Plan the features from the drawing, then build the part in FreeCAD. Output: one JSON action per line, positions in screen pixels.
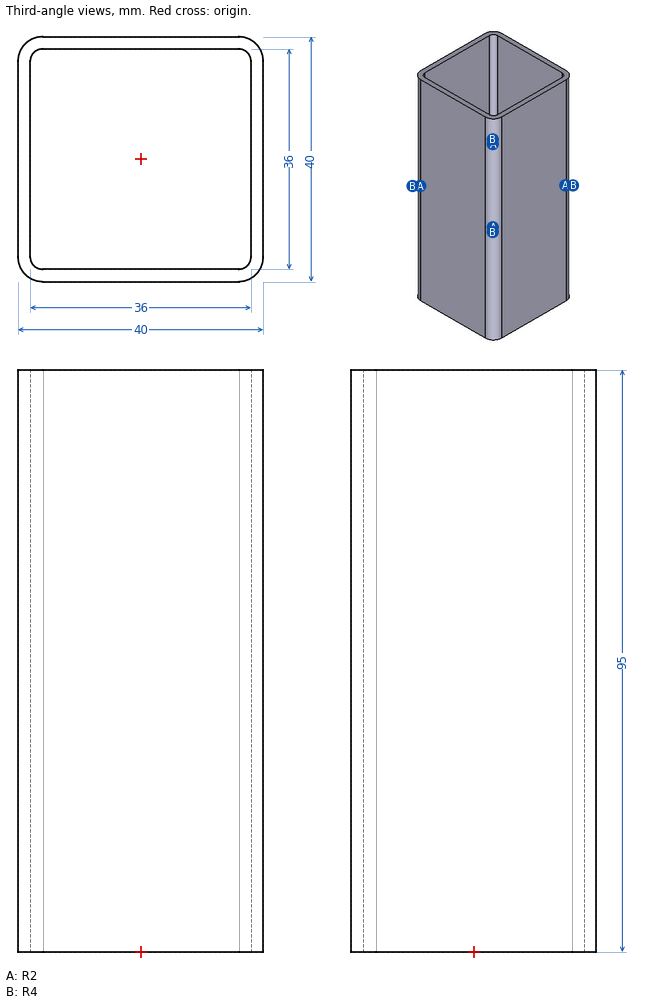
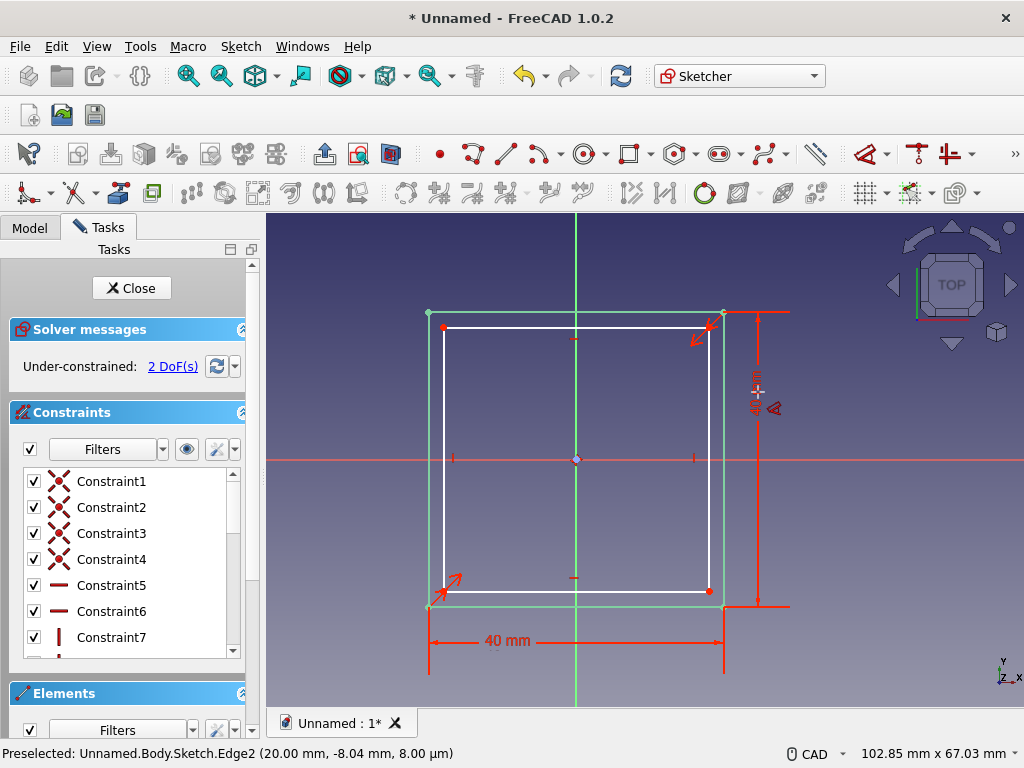
{"action": "left_click", "coordinate": [523, 592]}
{"action": "left_click", "coordinate": [637, 626]}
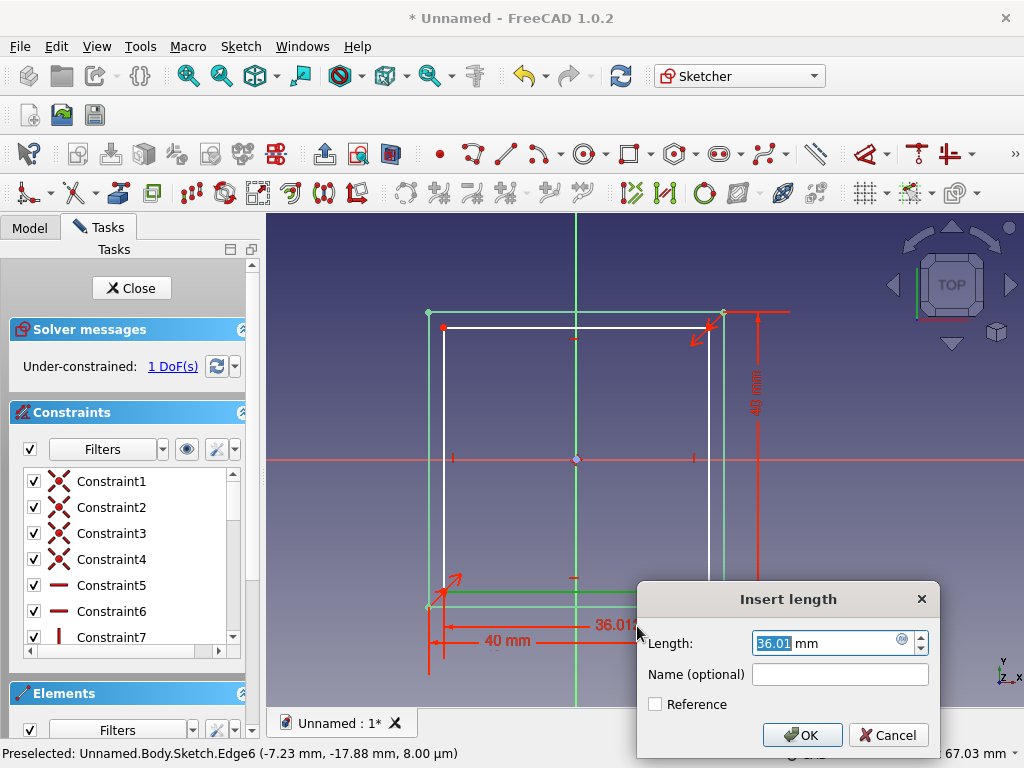
{"action": "type", "text": "36"}
{"action": "key", "text": "Return"}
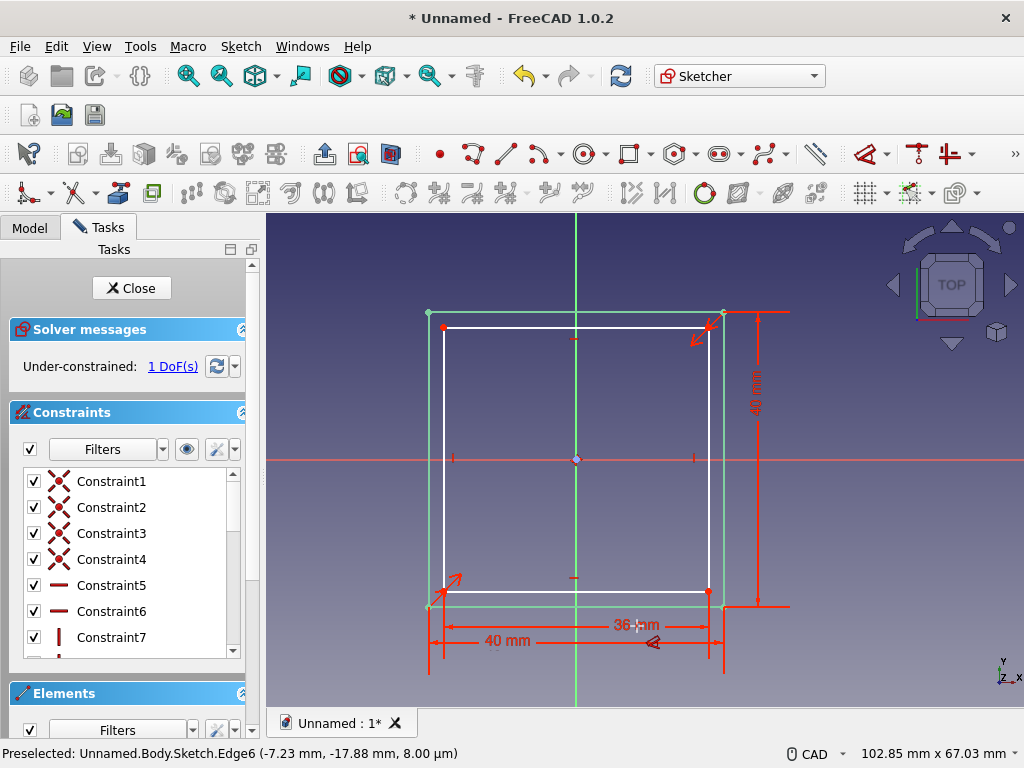
{"action": "left_click", "coordinate": [709, 512]}
{"action": "left_click", "coordinate": [743, 520]}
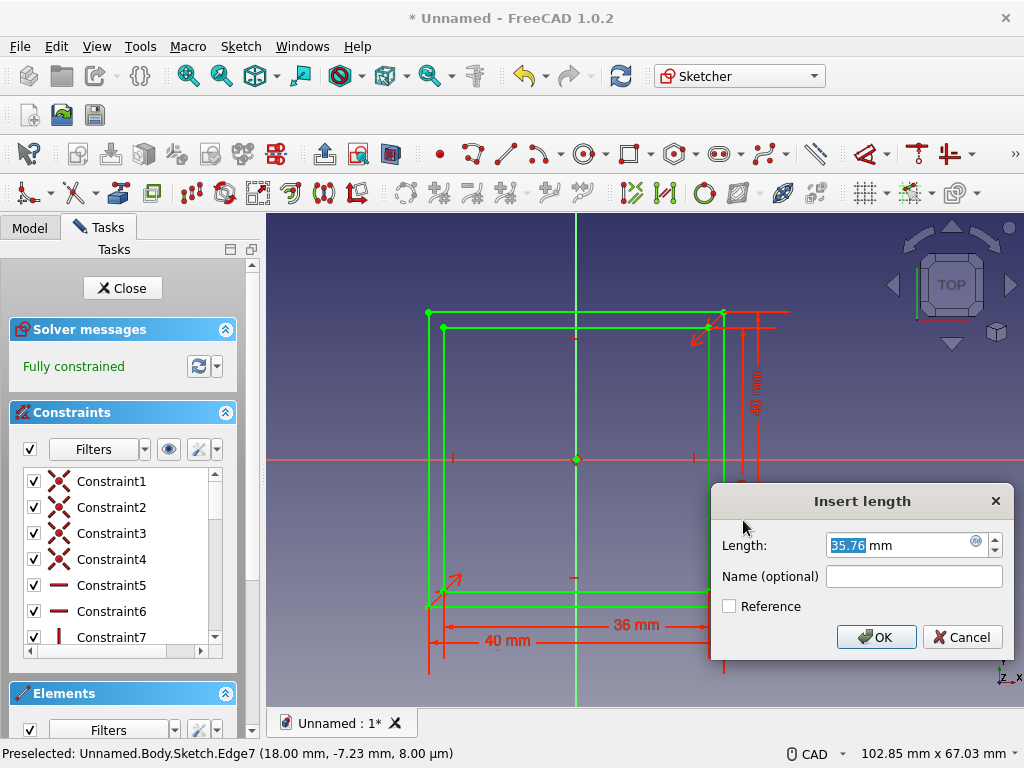
{"action": "type", "text": "36"}
{"action": "key", "text": "Return"}
{"action": "key", "text": "Escape"}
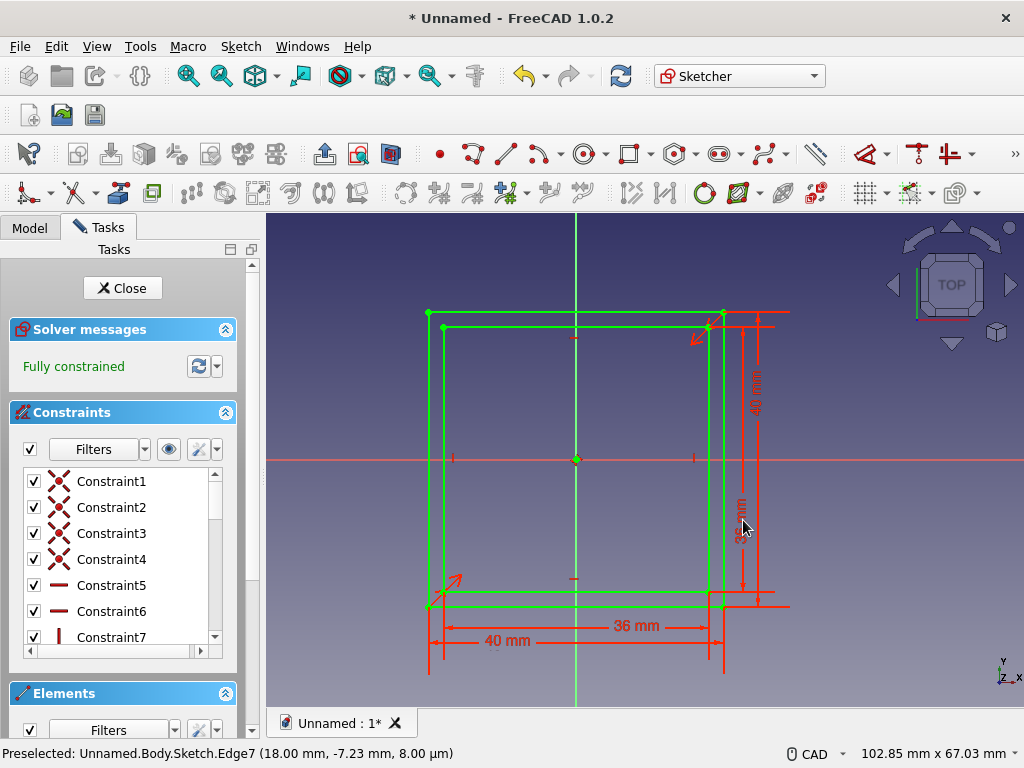
{"action": "left_click", "coordinate": [123, 288]}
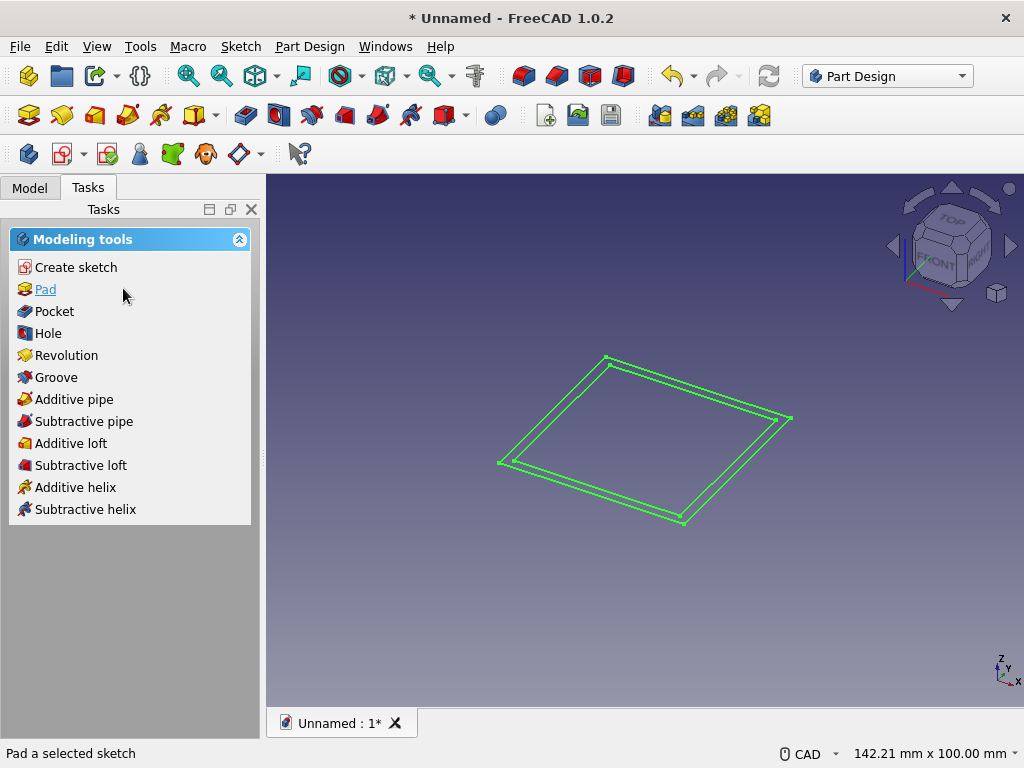
{"action": "left_click", "coordinate": [29, 116]}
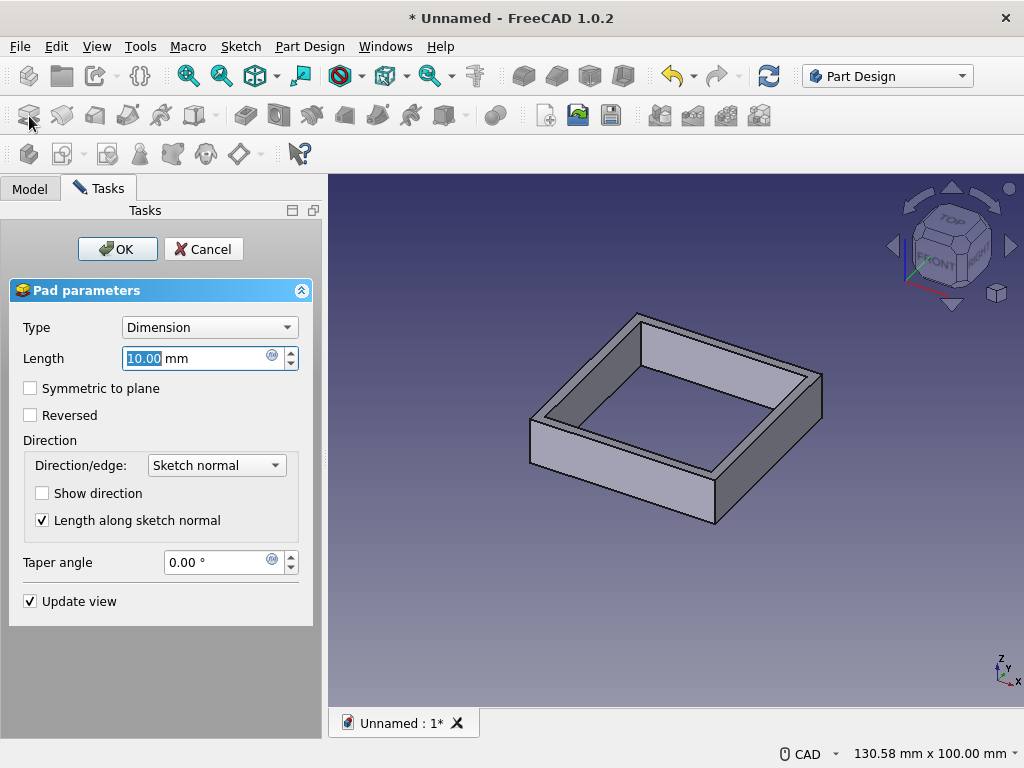
{"action": "type", "text": "95"}
{"action": "key", "text": "Tab"}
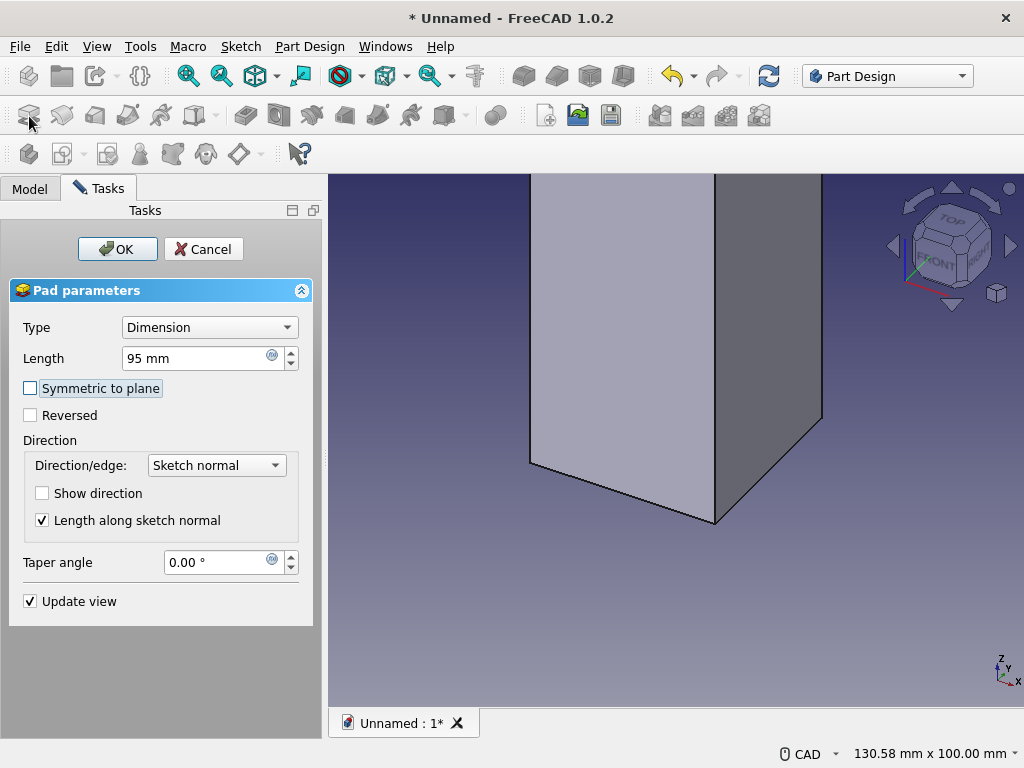
{"action": "left_click", "coordinate": [118, 249]}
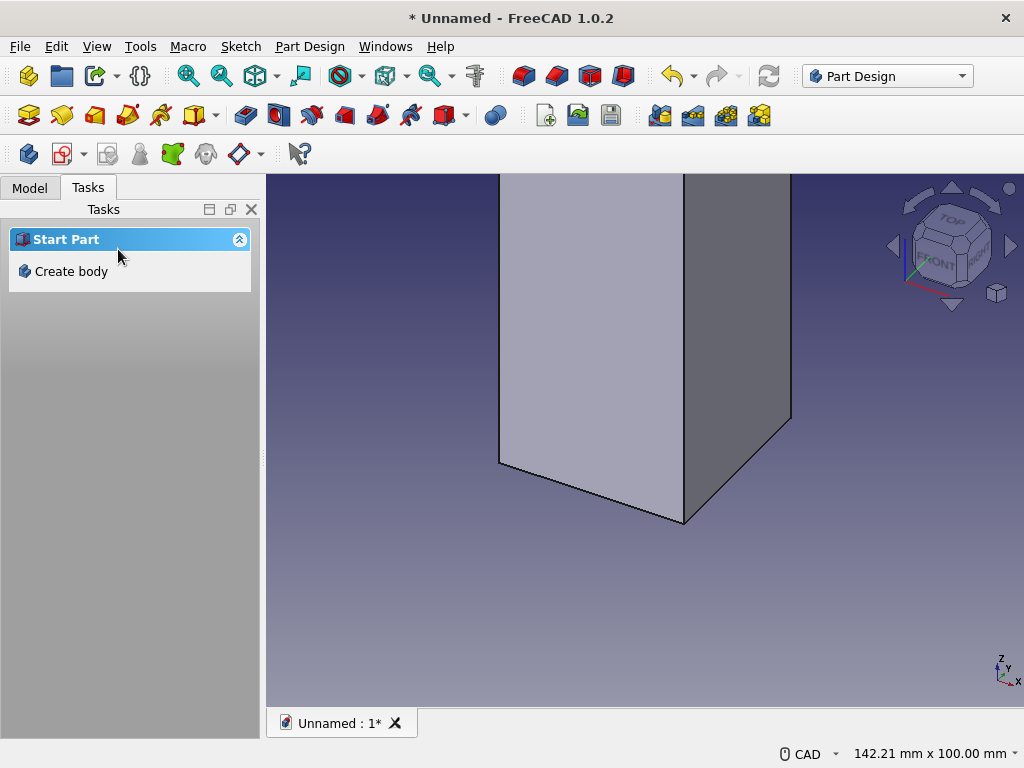
{"action": "left_click", "coordinate": [189, 76]}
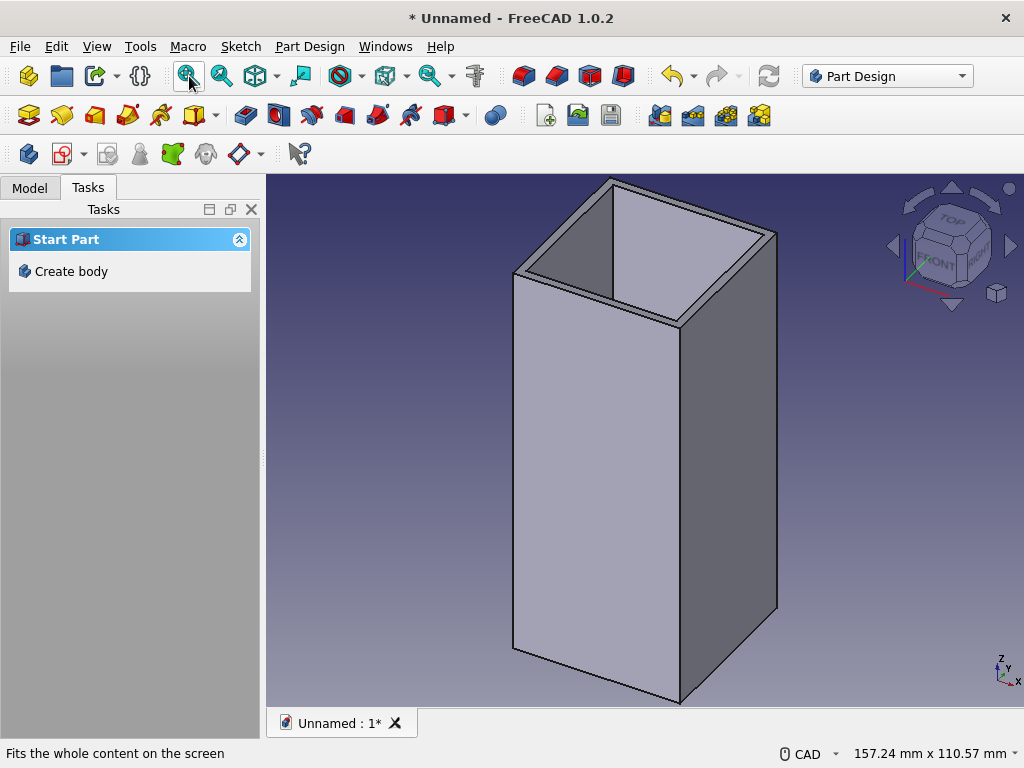
{"action": "key", "text": "0"}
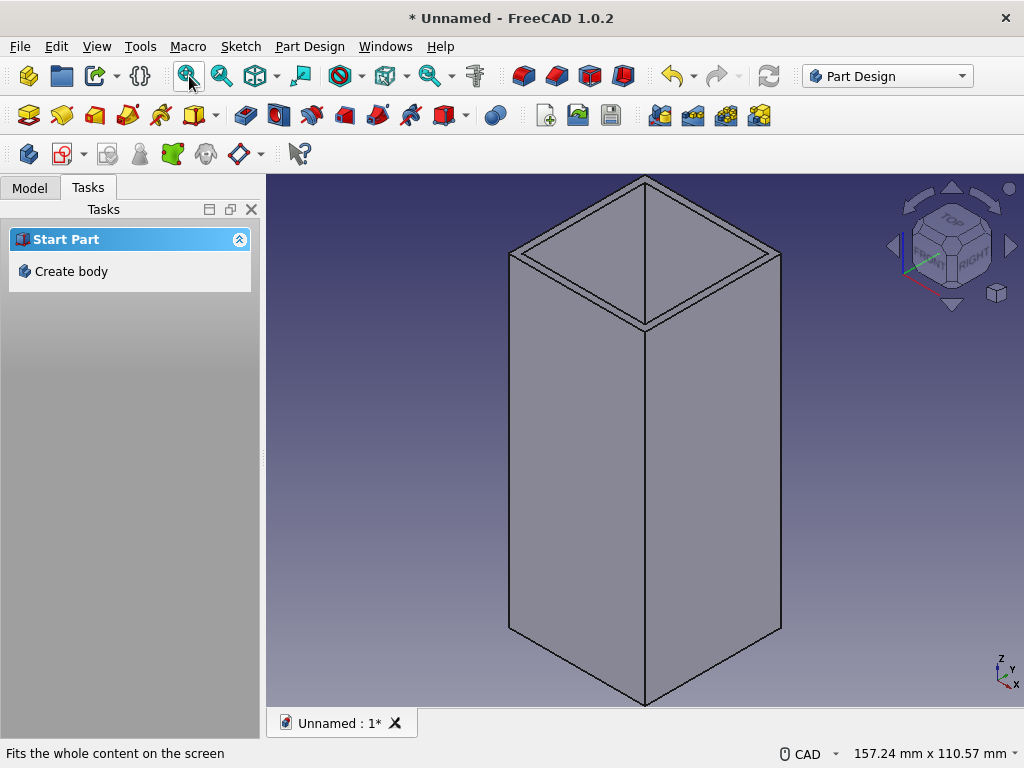
{"action": "key", "text": "2"}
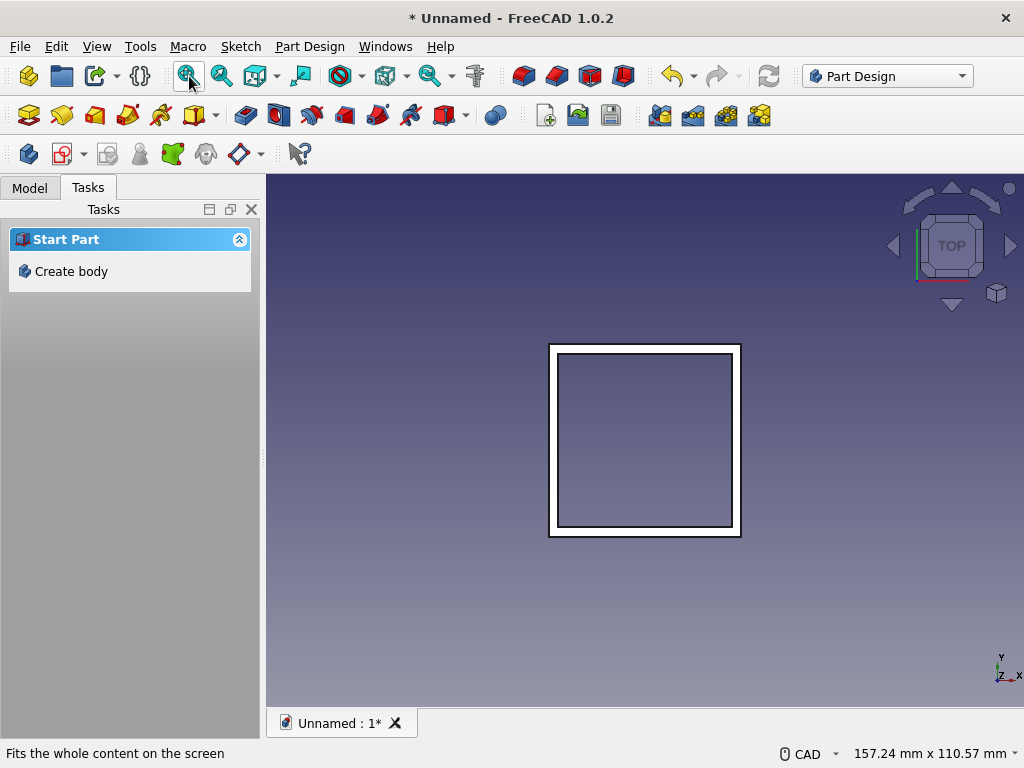
{"action": "left_click", "coordinate": [189, 76]}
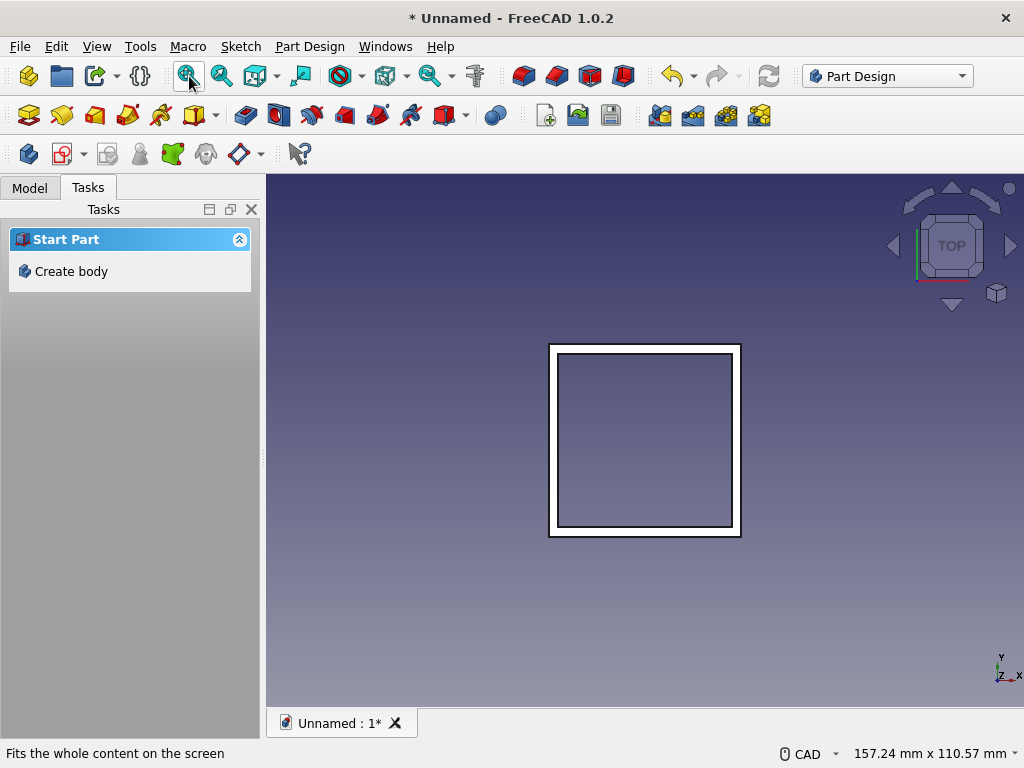
{"action": "key", "text": "1"}